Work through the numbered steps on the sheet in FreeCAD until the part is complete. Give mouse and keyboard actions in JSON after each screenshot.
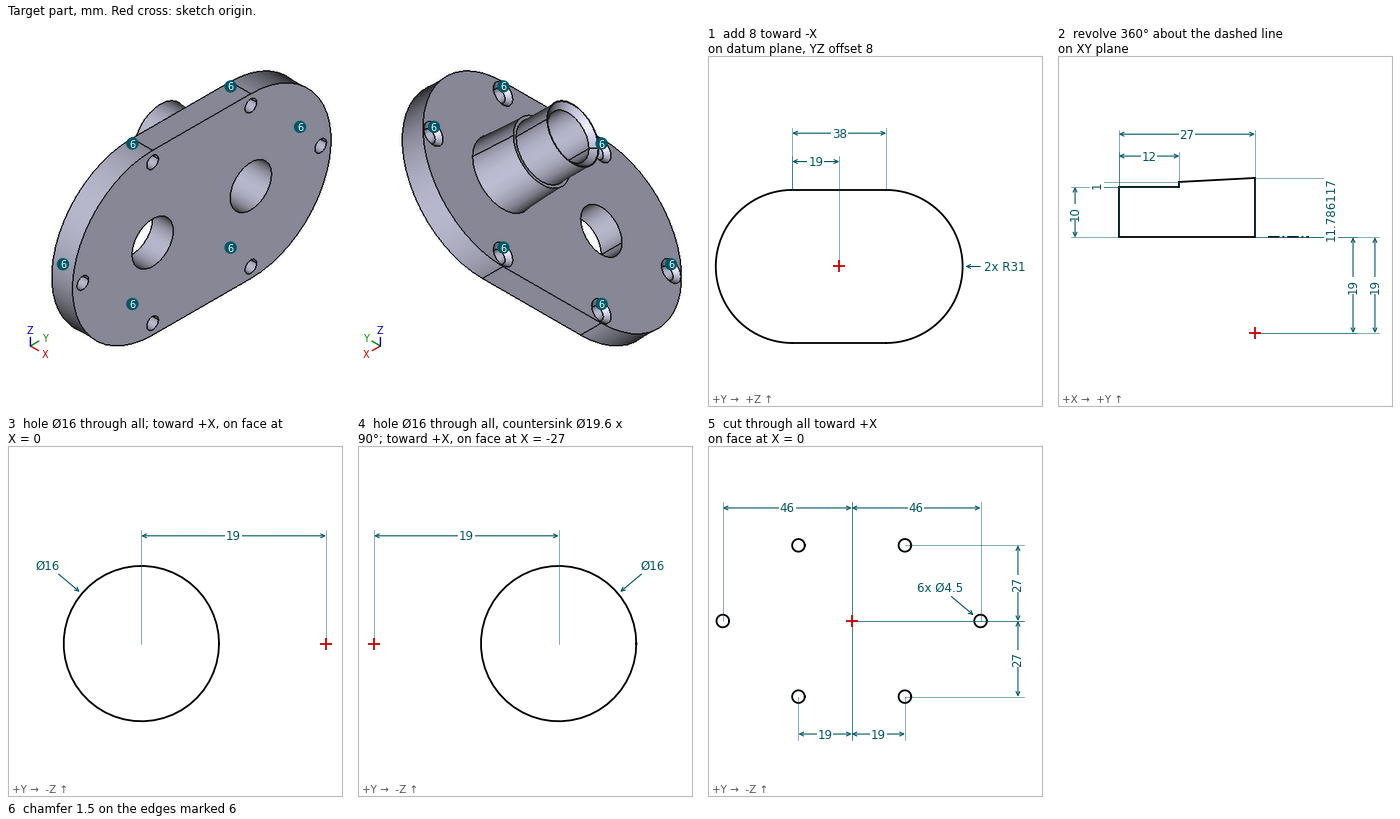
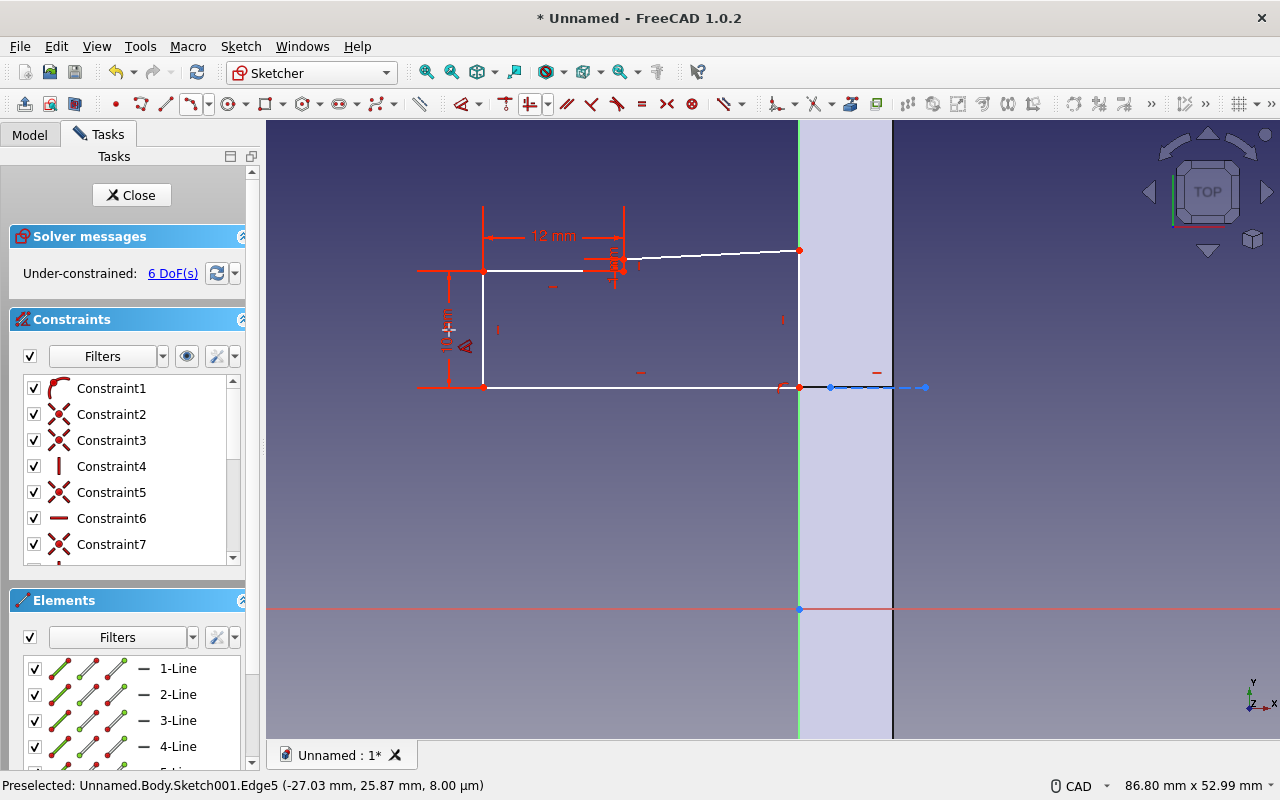
{"action": "left_click", "coordinate": [578, 388]}
{"action": "left_click", "coordinate": [641, 354]}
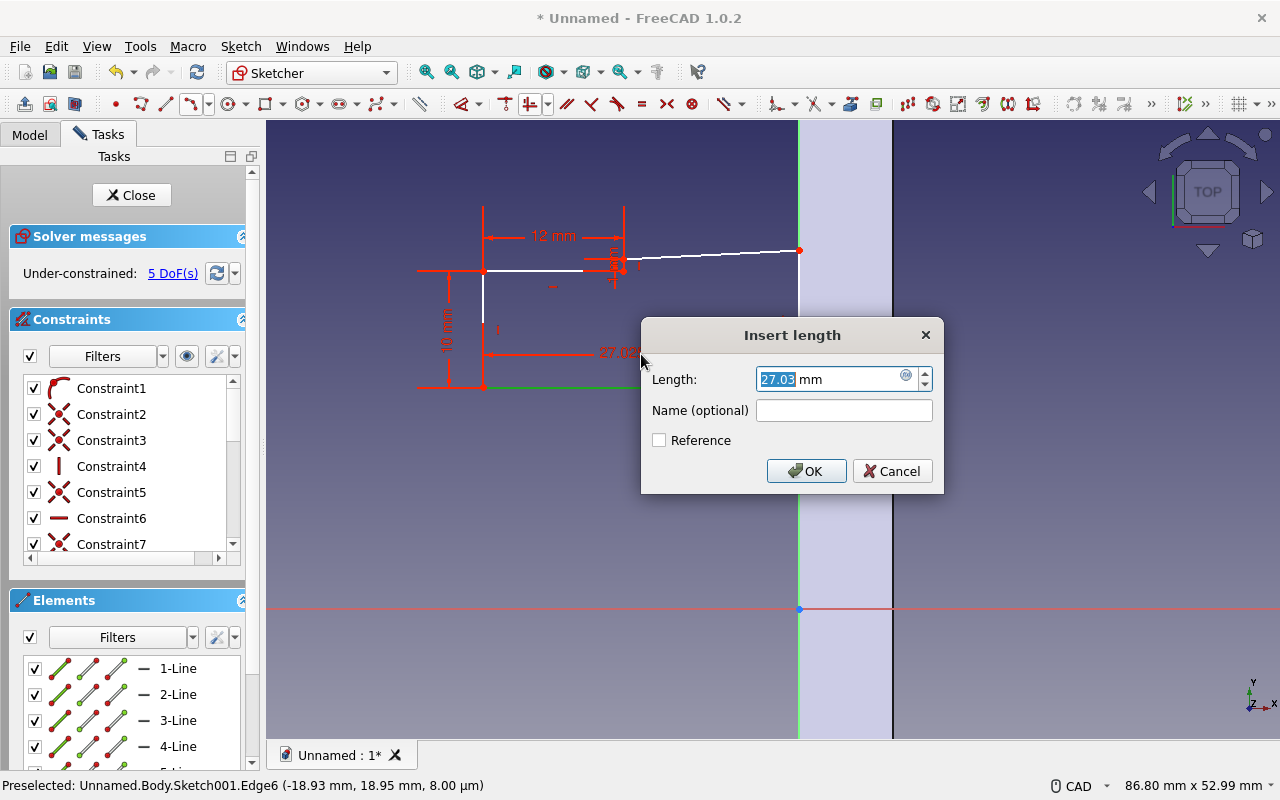
{"action": "type", "text": "27"}
{"action": "key", "text": "Return"}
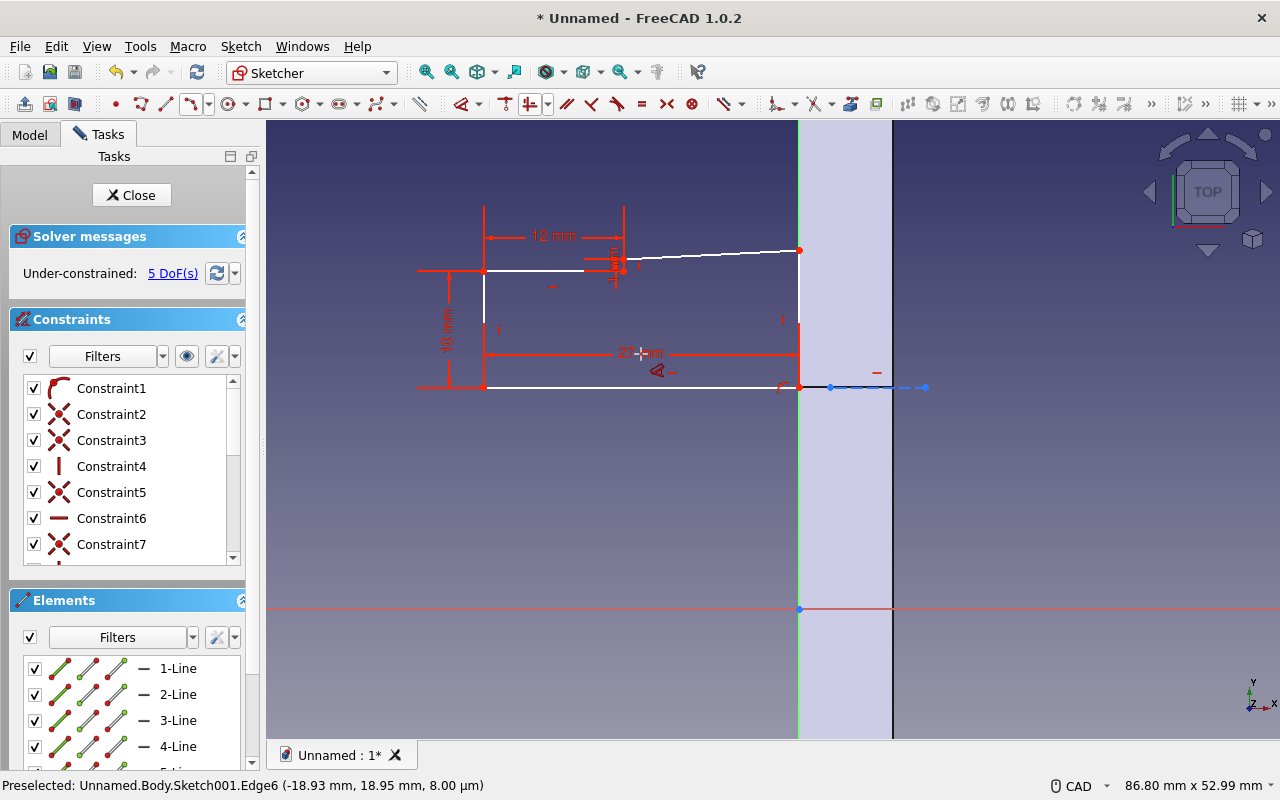
{"action": "left_click", "coordinate": [799, 388]}
{"action": "left_click", "coordinate": [833, 499]}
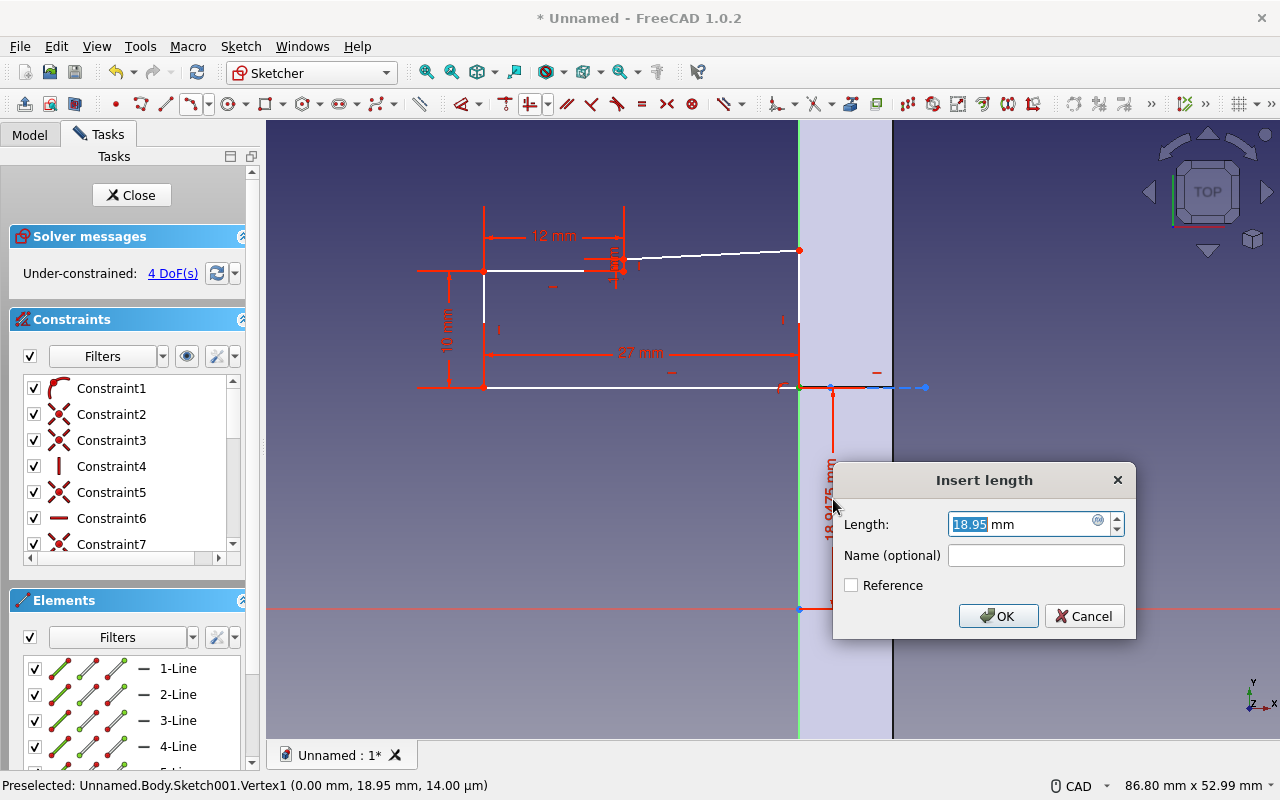
{"action": "type", "text": "19"}
{"action": "key", "text": "Return"}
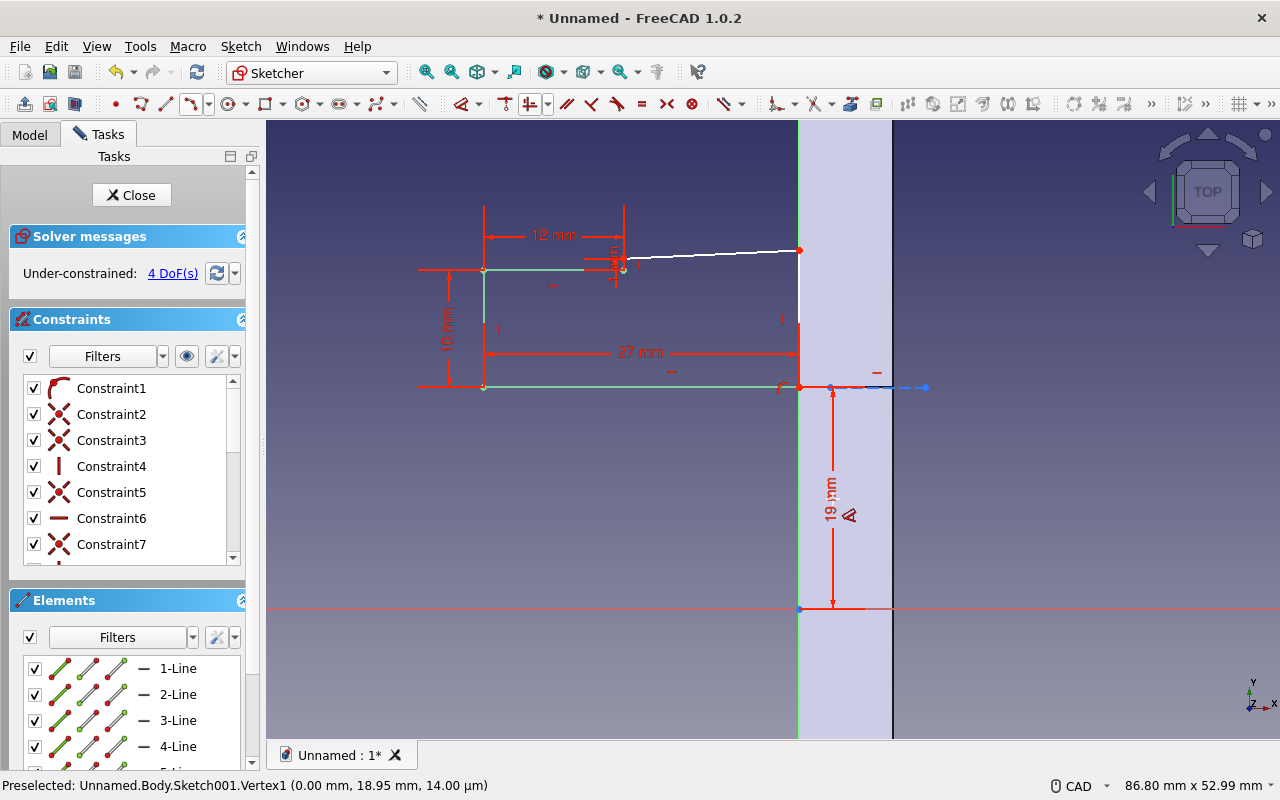
{"action": "left_click", "coordinate": [831, 388]}
{"action": "left_click", "coordinate": [865, 448]}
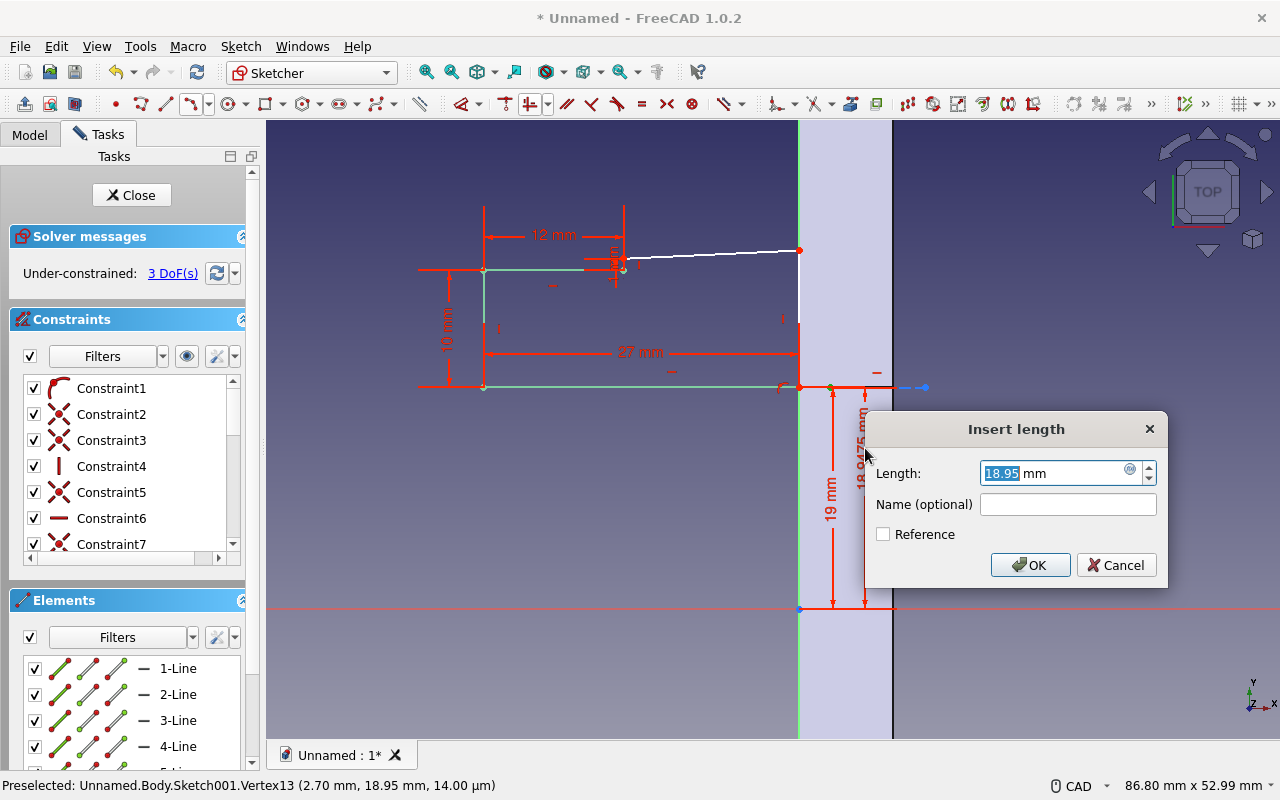
{"action": "type", "text": "19"}
{"action": "key", "text": "Return"}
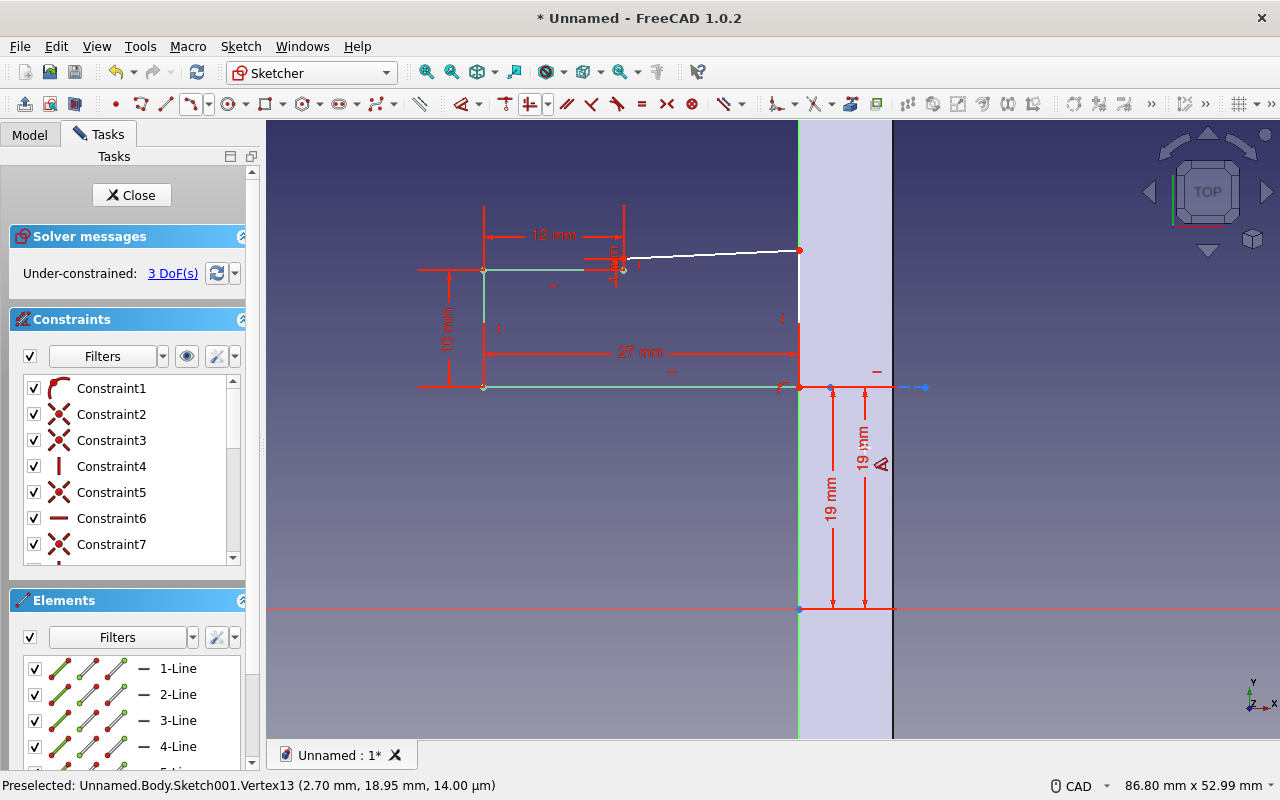
{"action": "left_click", "coordinate": [799, 346]}
{"action": "left_click", "coordinate": [833, 319]}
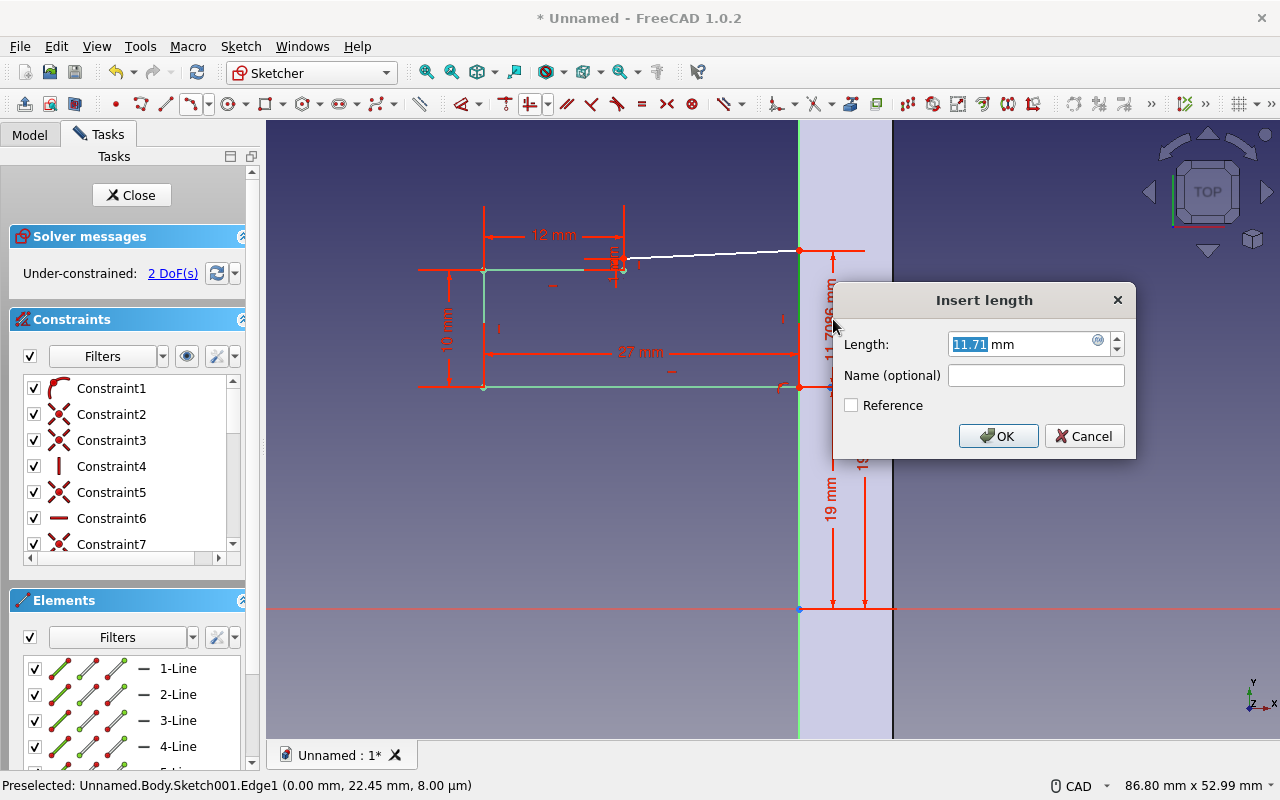
{"action": "type", "text": "11.786117"}
{"action": "key", "text": "Return"}
{"action": "key", "text": "Escape"}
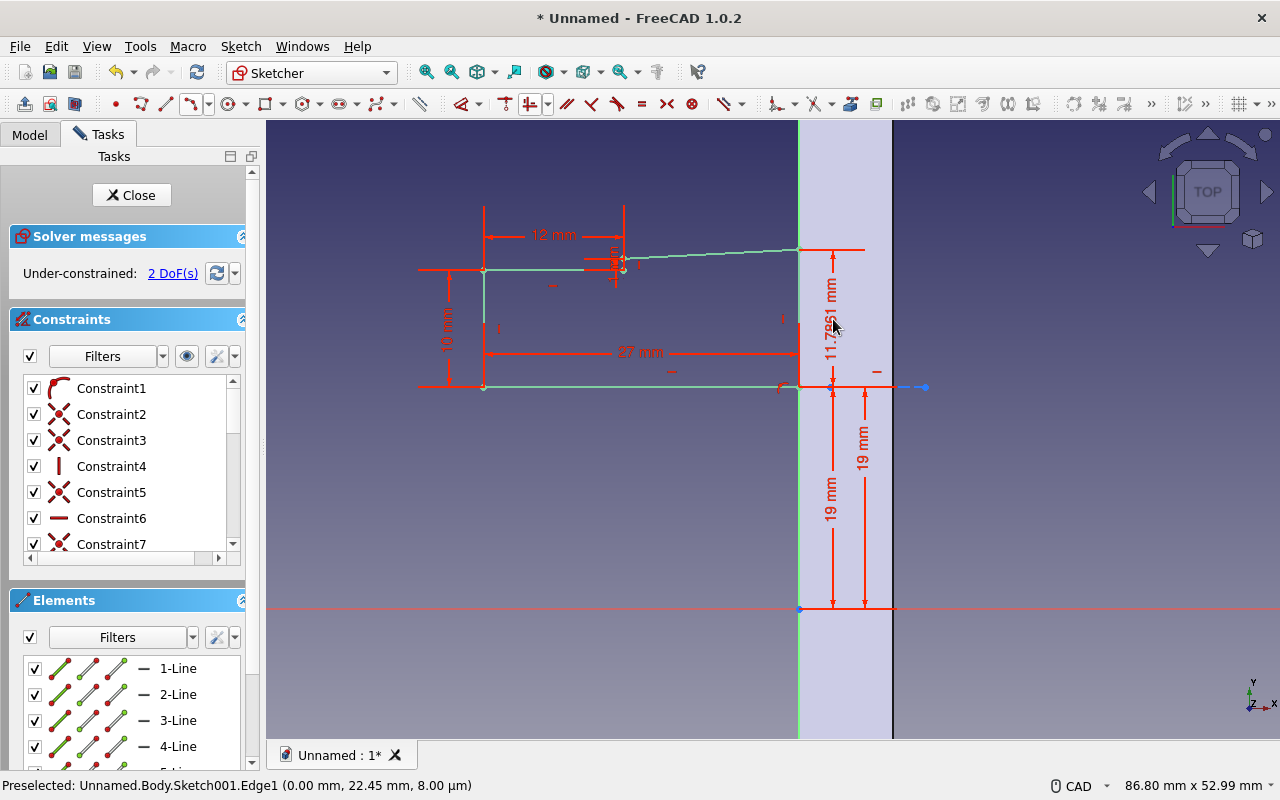
{"action": "left_click", "coordinate": [132, 195]}